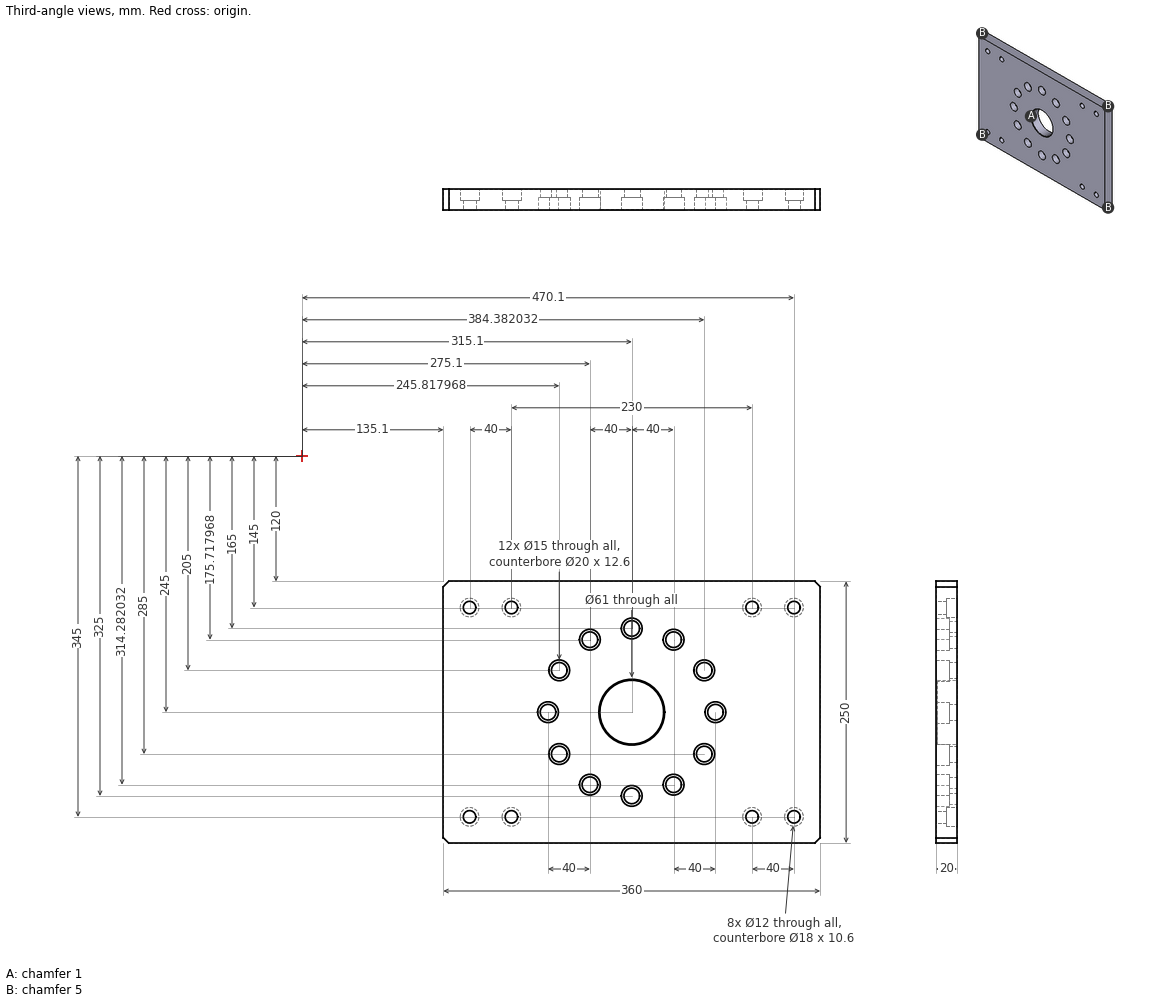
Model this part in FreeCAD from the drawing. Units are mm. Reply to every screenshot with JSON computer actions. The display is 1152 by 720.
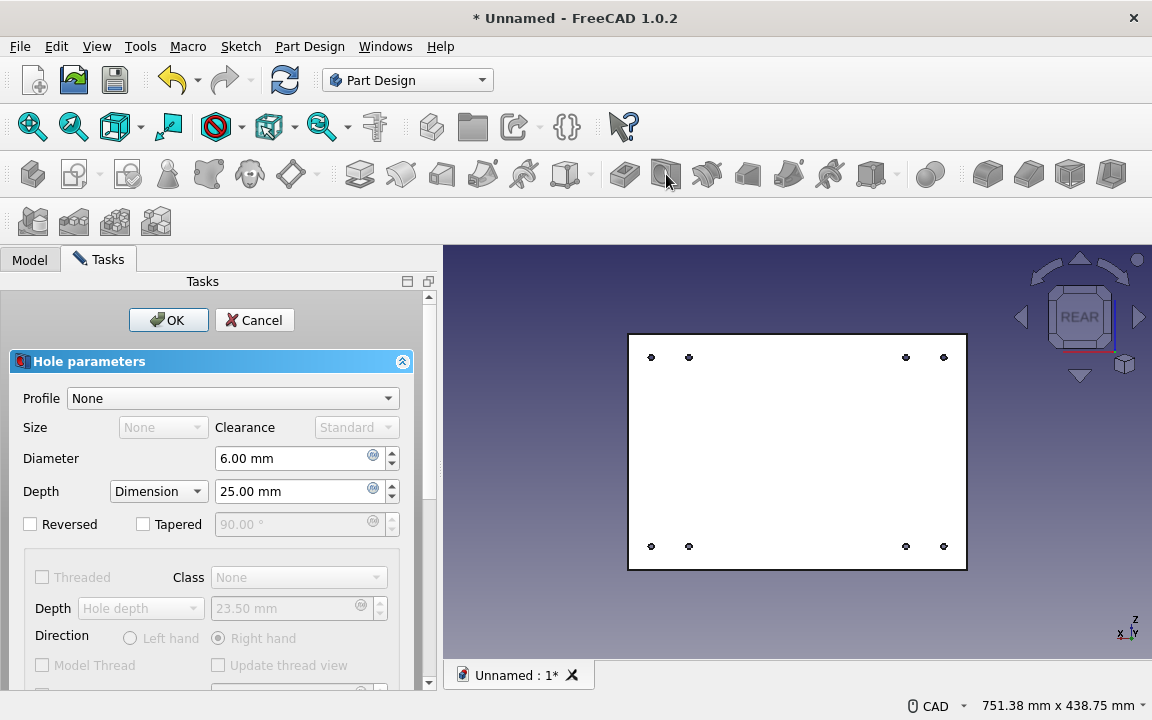
{"action": "triple_click", "coordinate": [300, 458]}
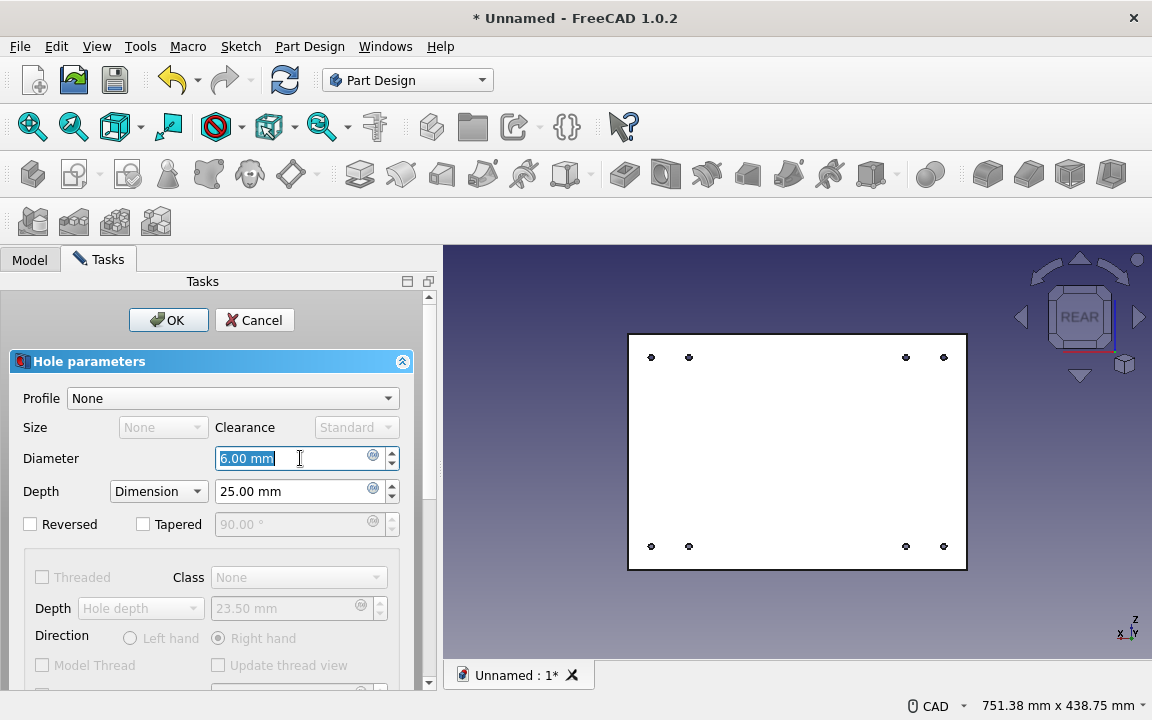
{"action": "type", "text": "12"}
{"action": "key", "text": "Tab"}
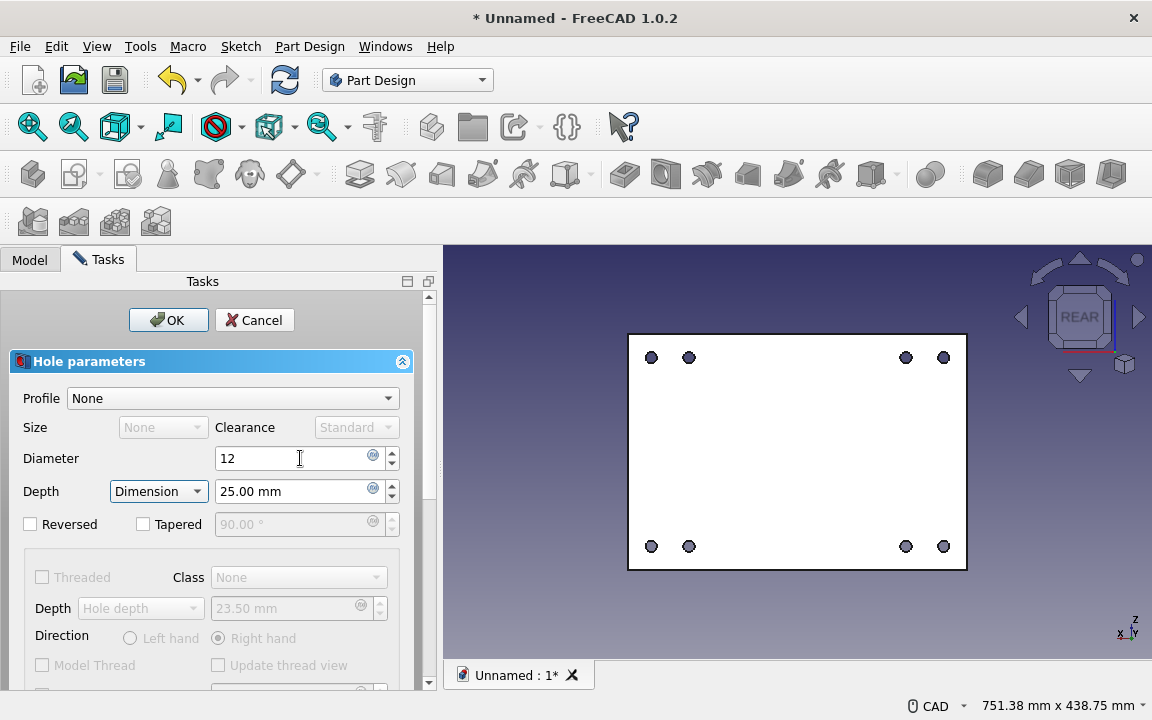
{"action": "left_click", "coordinate": [160, 492]}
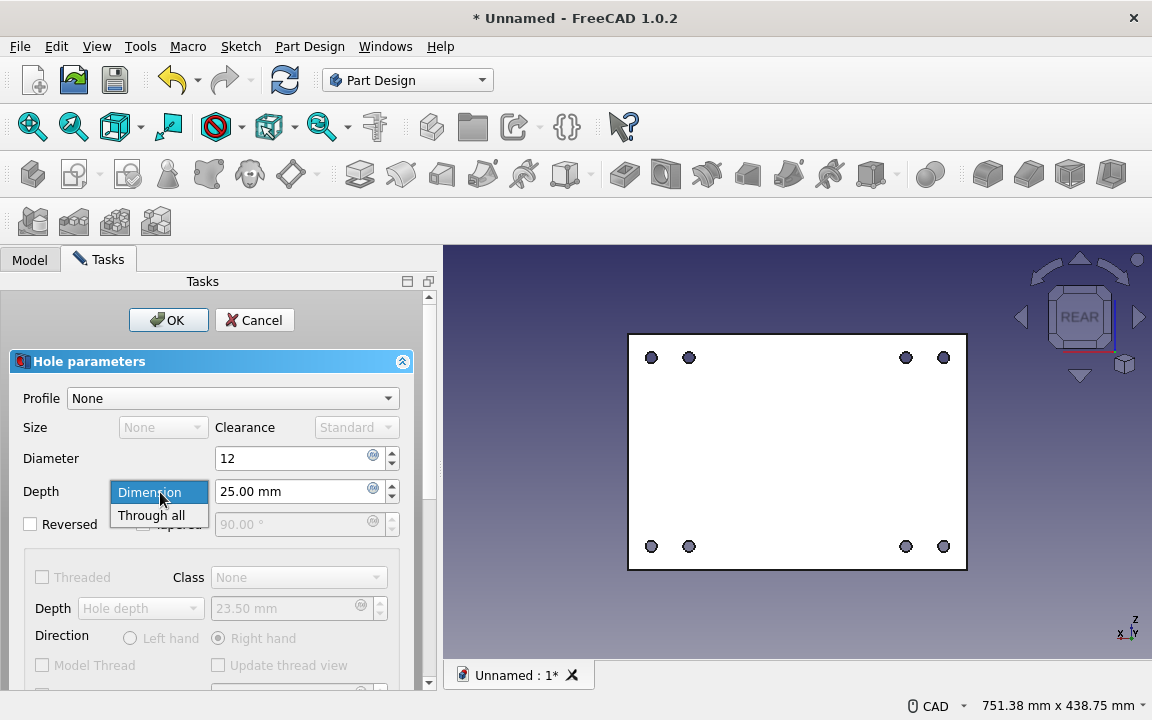
{"action": "left_click", "coordinate": [158, 516]}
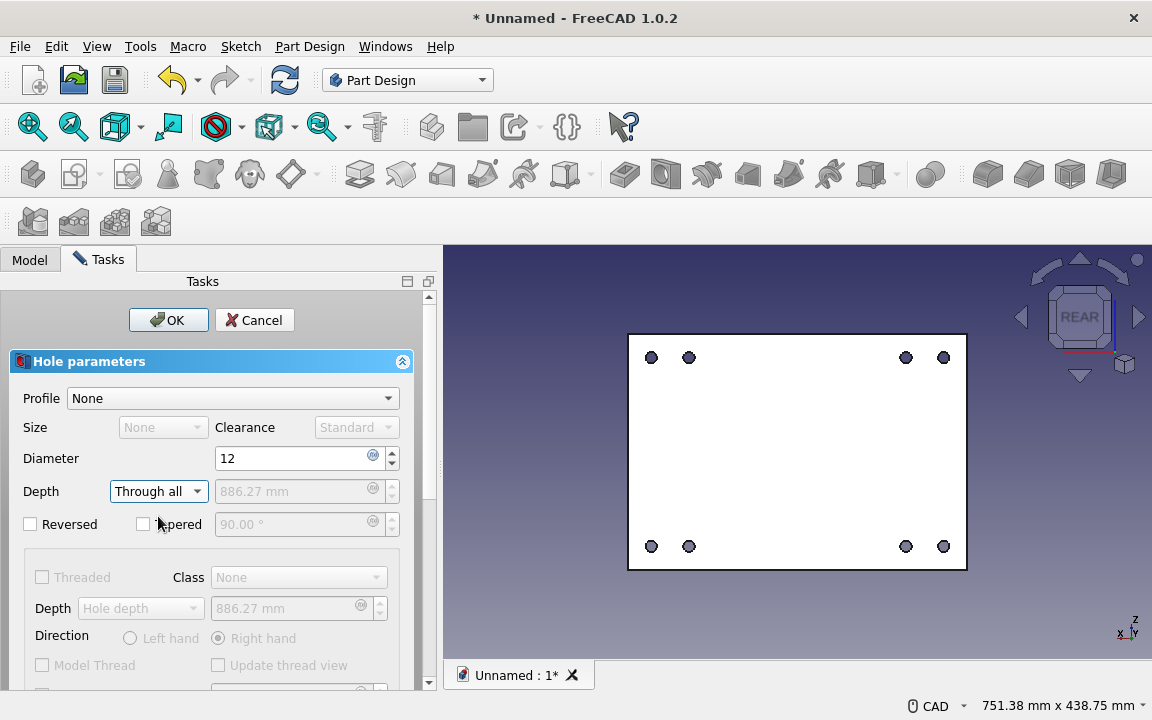
{"action": "scroll", "coordinate": [429, 490], "scroll_direction": "down", "scroll_amount": 3}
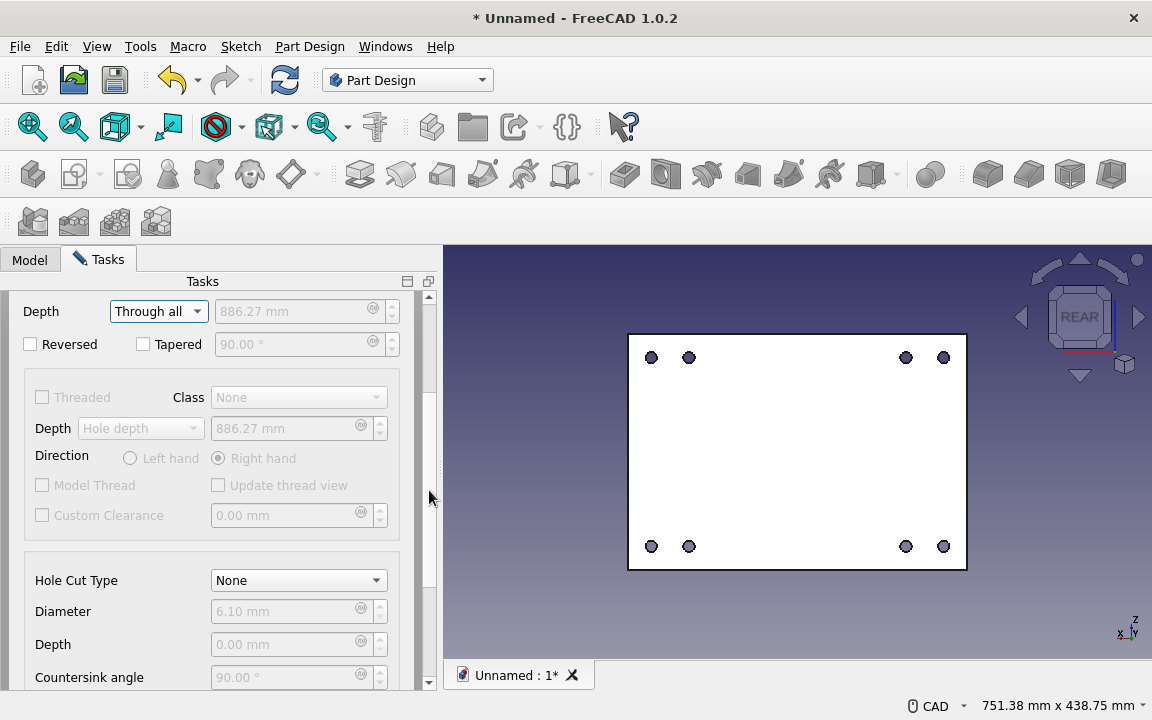
{"action": "left_click", "coordinate": [300, 580]}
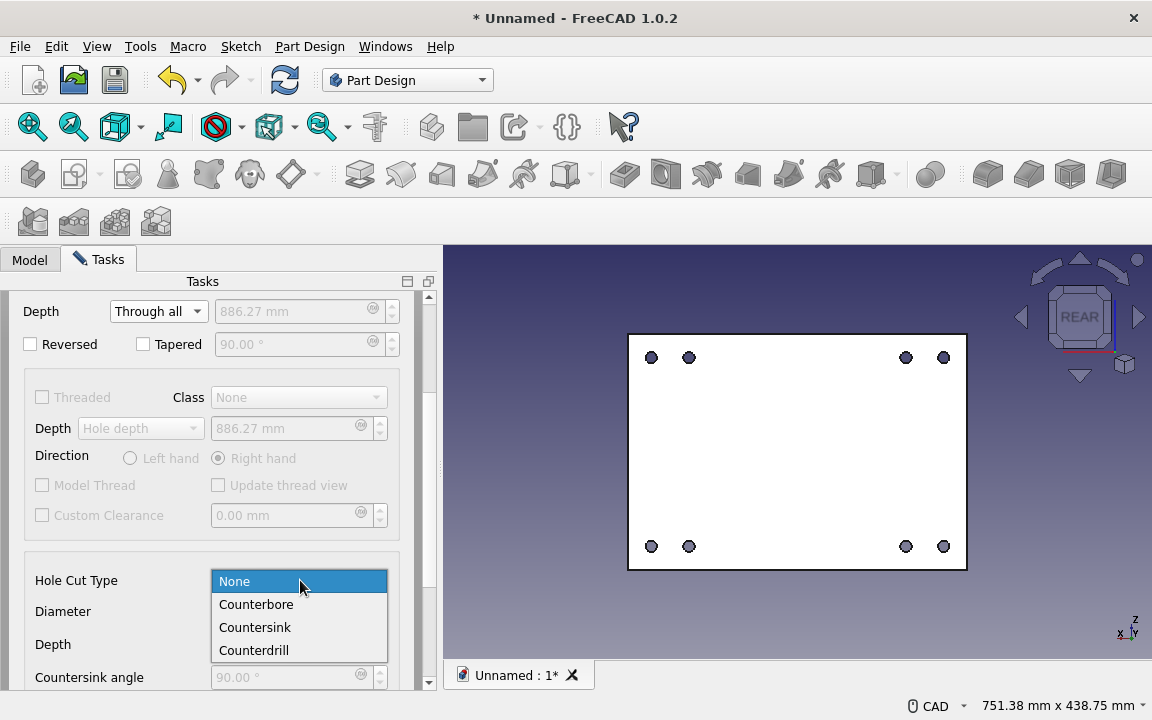
{"action": "left_click", "coordinate": [298, 604]}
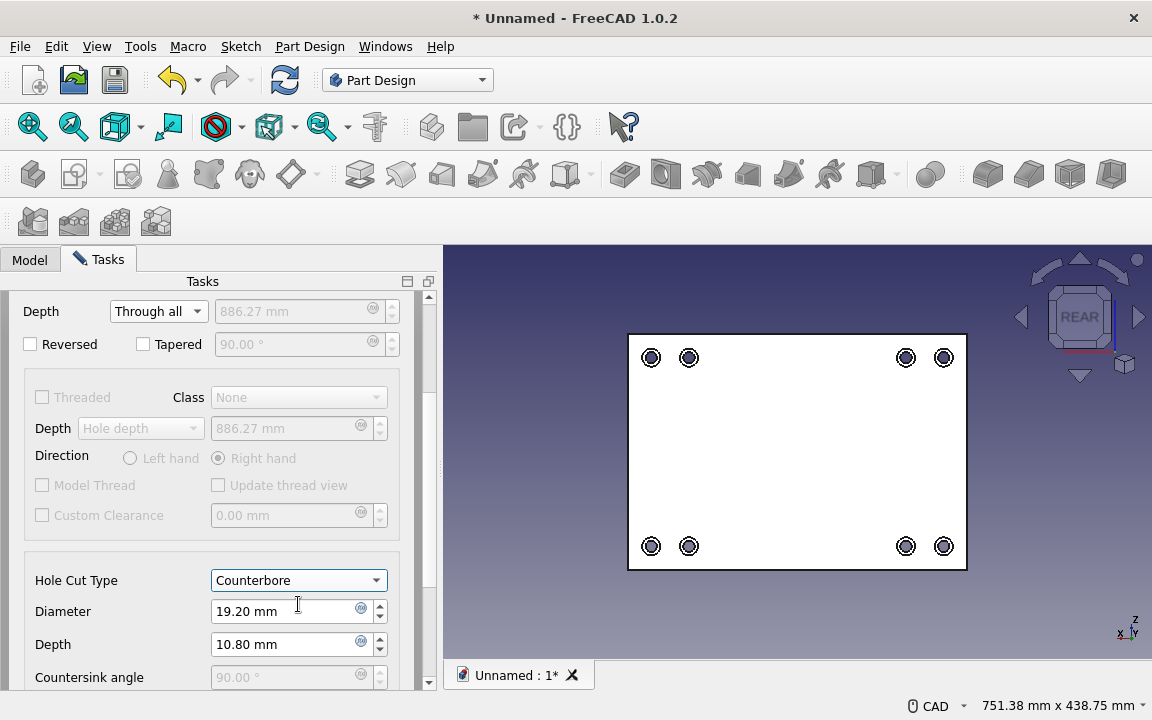
{"action": "triple_click", "coordinate": [292, 612]}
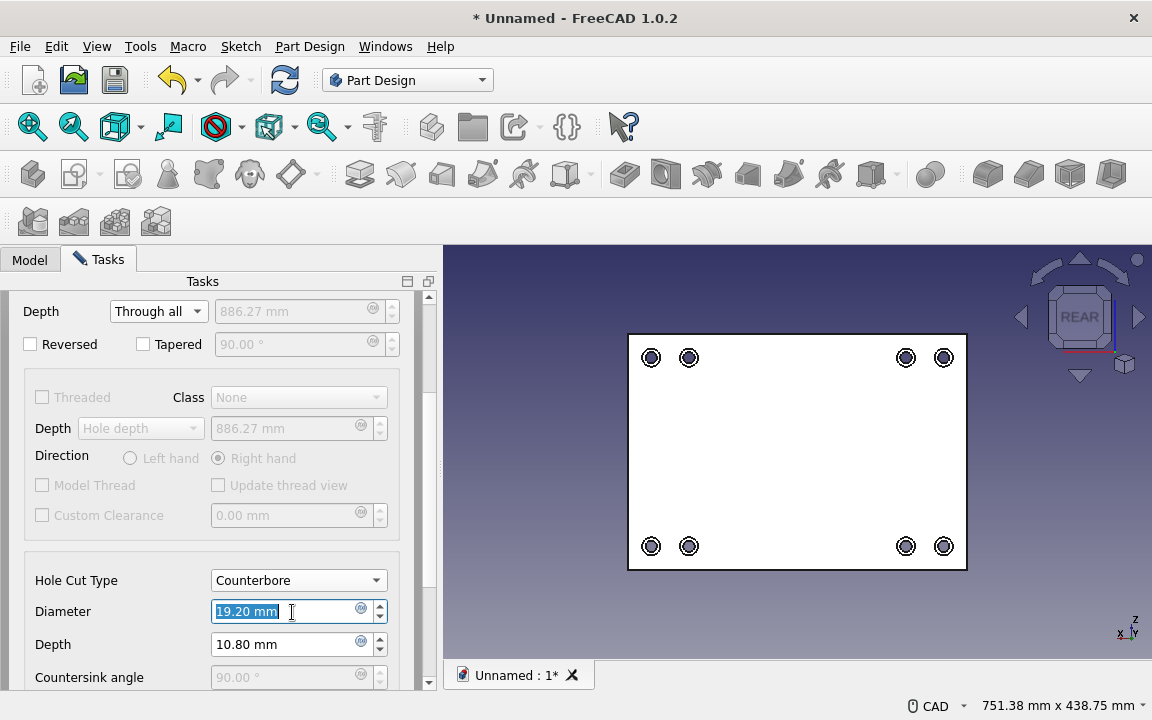
{"action": "type", "text": "18"}
{"action": "key", "text": "Tab"}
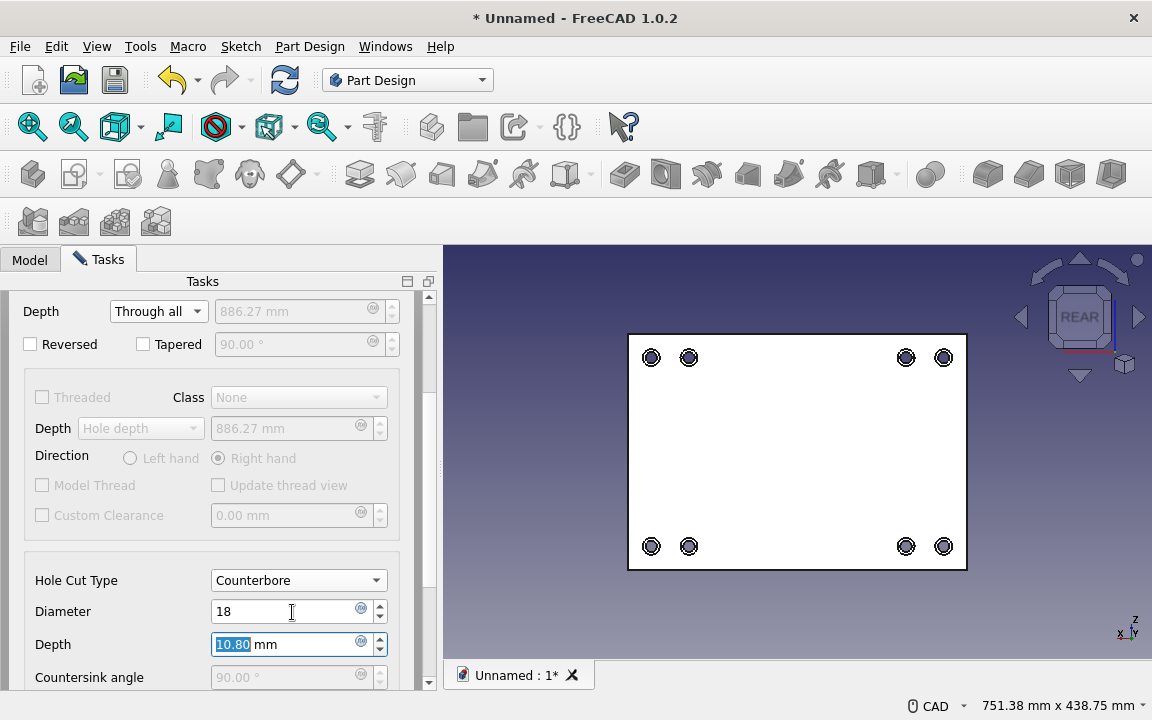
{"action": "type", "text": "10.6"}
{"action": "key", "text": "Tab"}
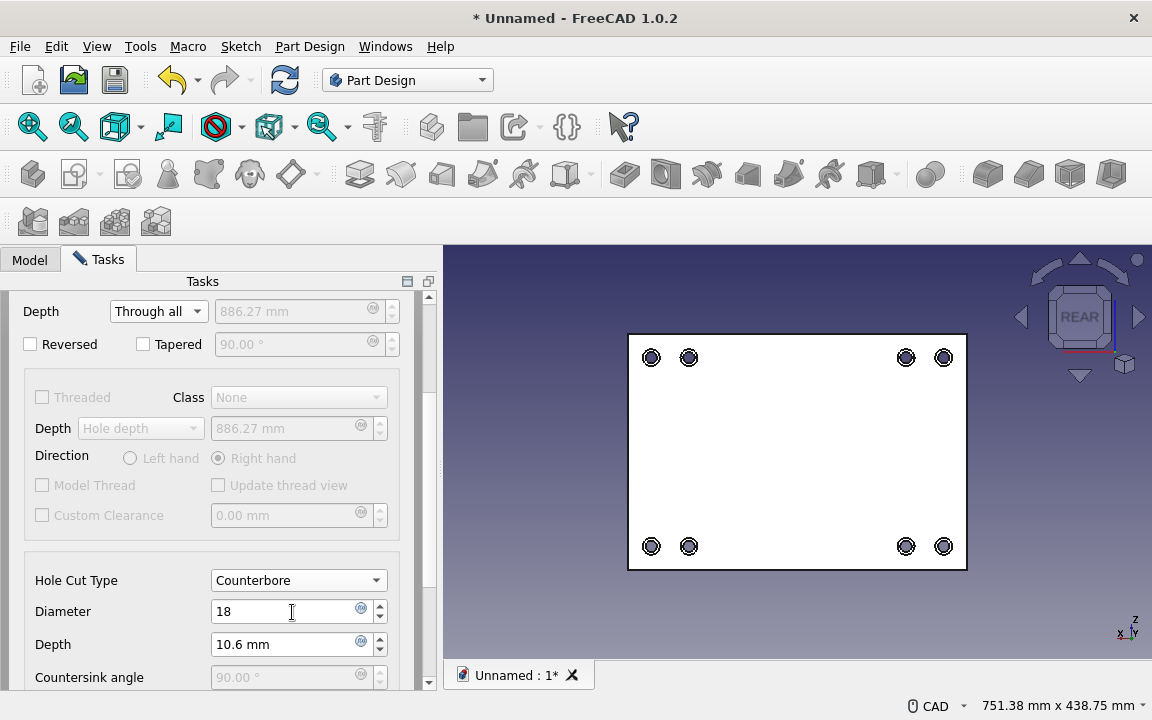
{"action": "scroll", "coordinate": [429, 490], "scroll_direction": "up", "scroll_amount": 4}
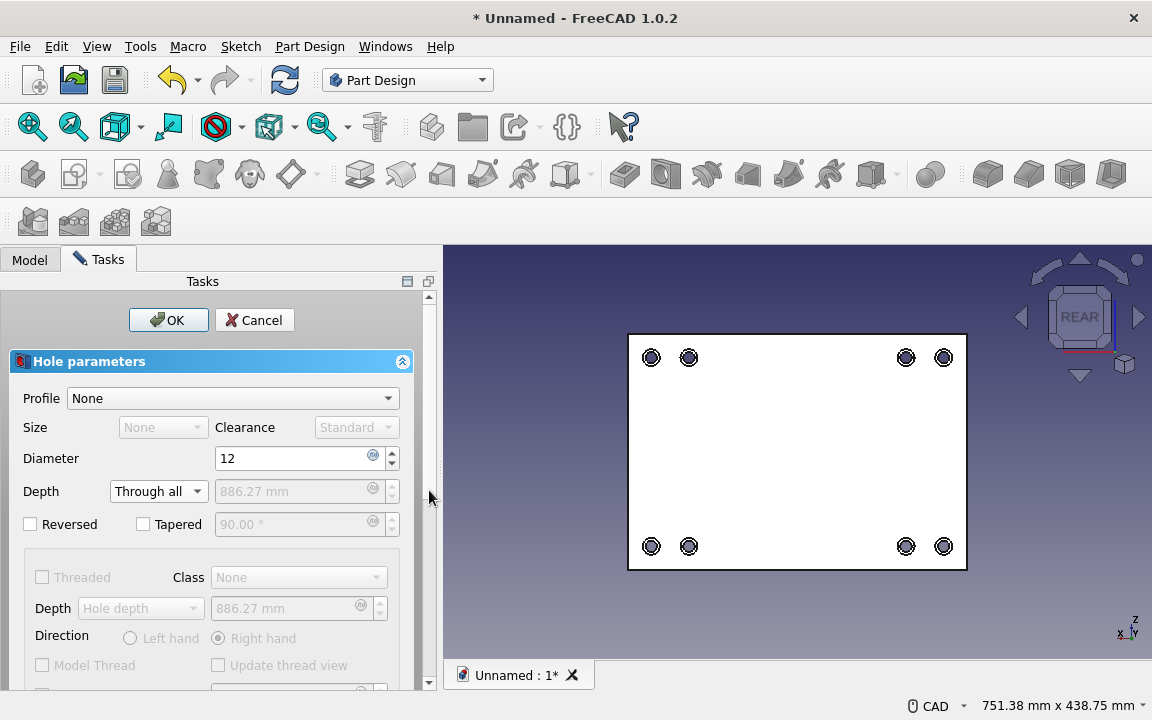
{"action": "left_click", "coordinate": [169, 320]}